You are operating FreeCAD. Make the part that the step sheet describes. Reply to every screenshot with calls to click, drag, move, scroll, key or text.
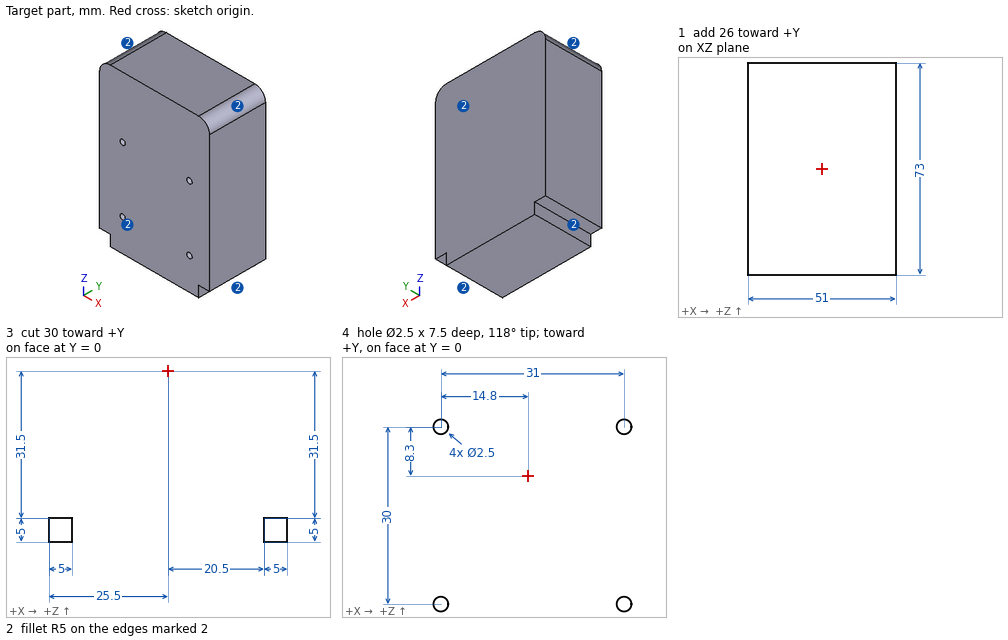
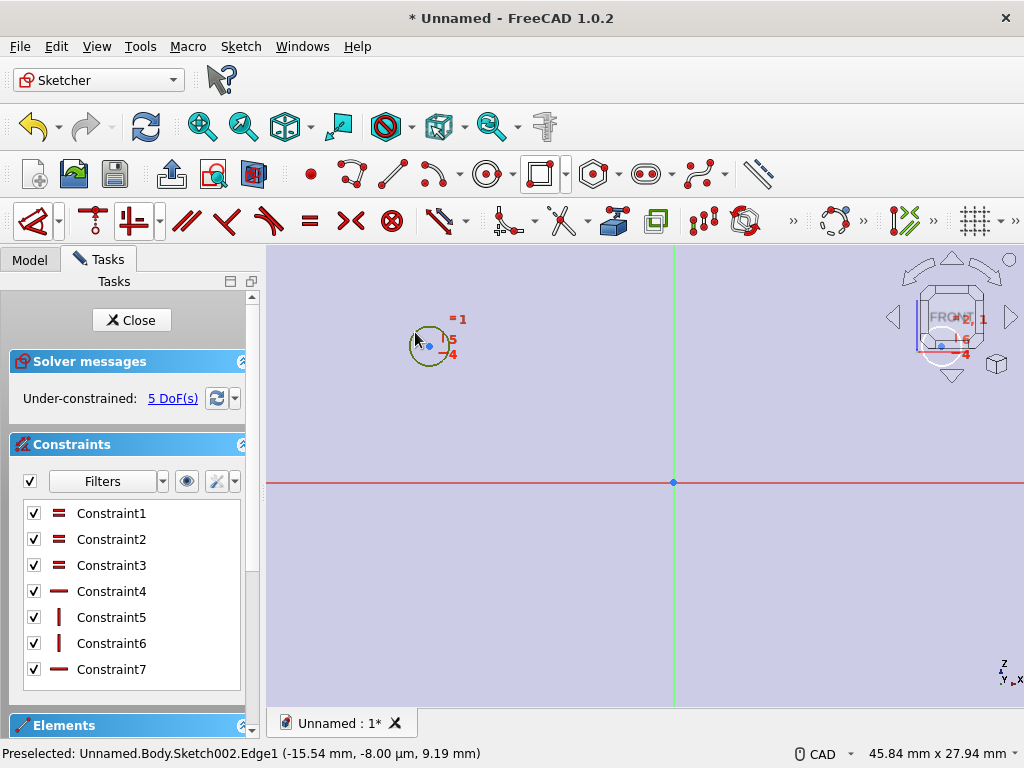
click(58, 222)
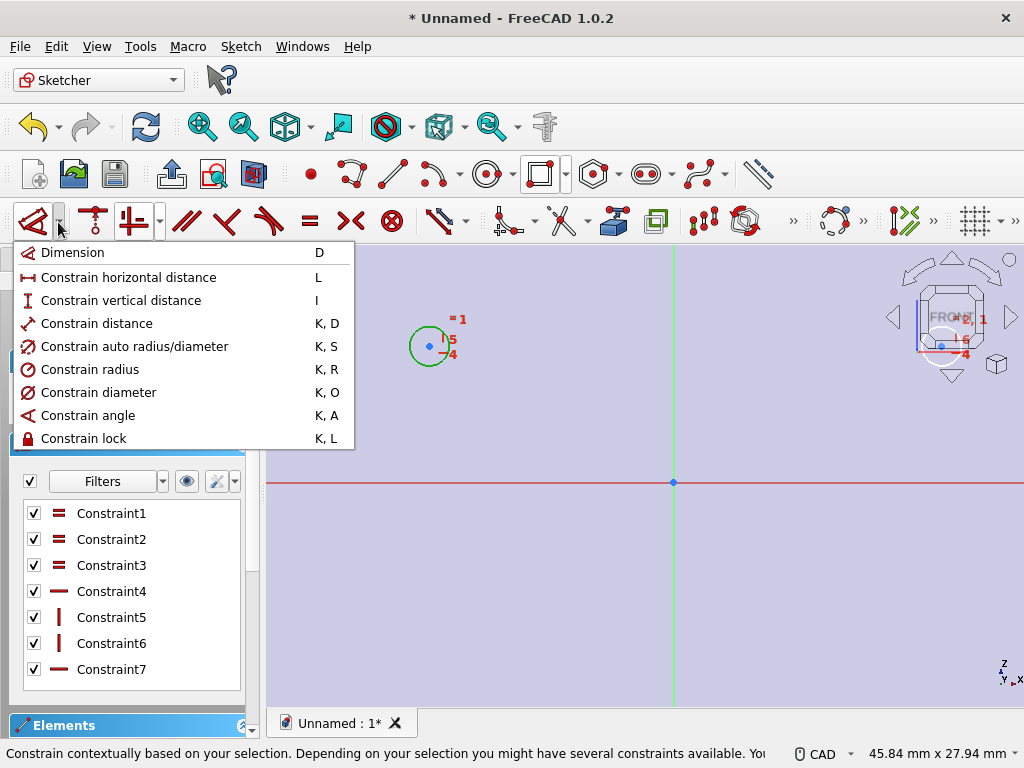
click(184, 392)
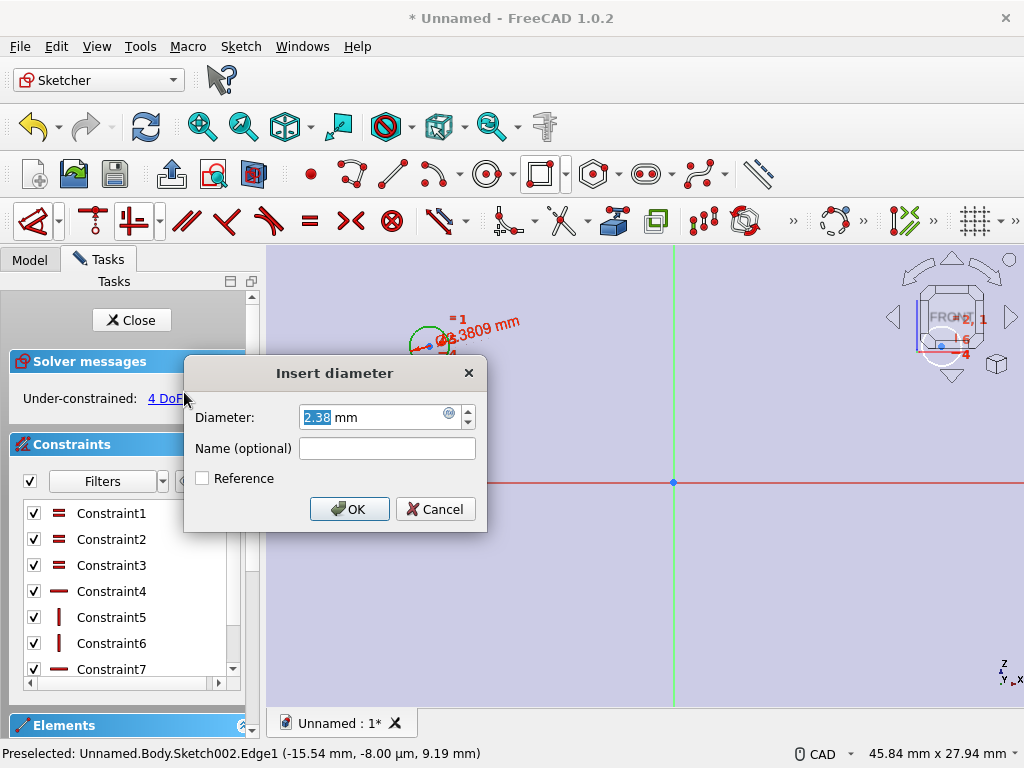
text(2.5)
key(Return)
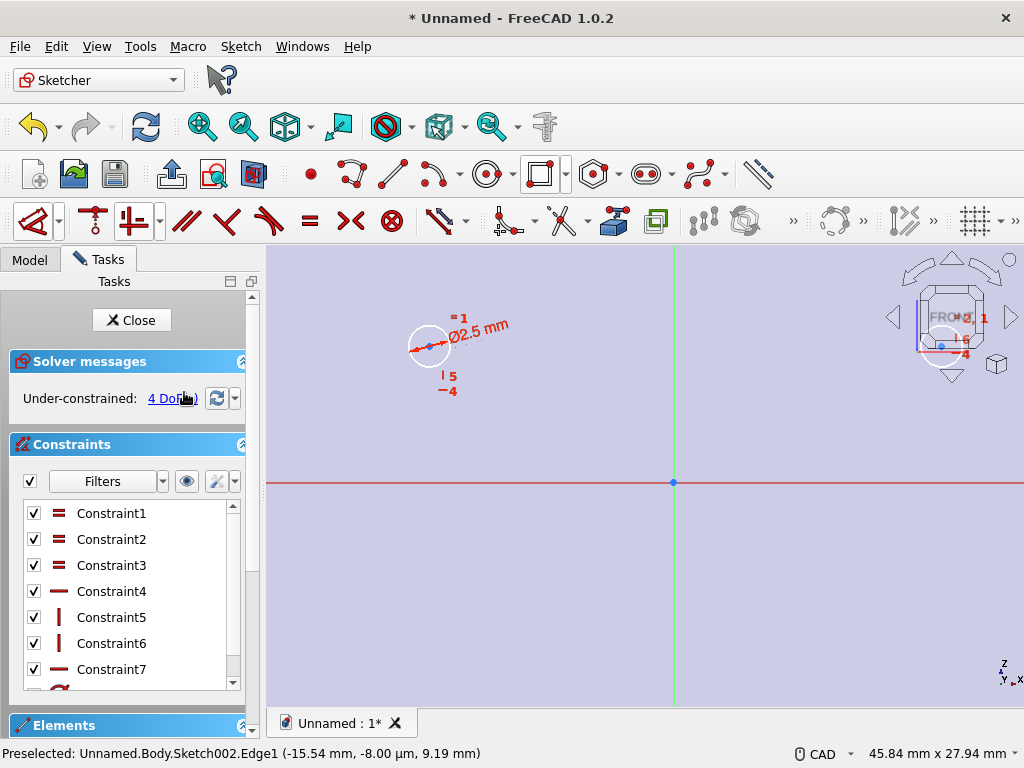
click(429, 346)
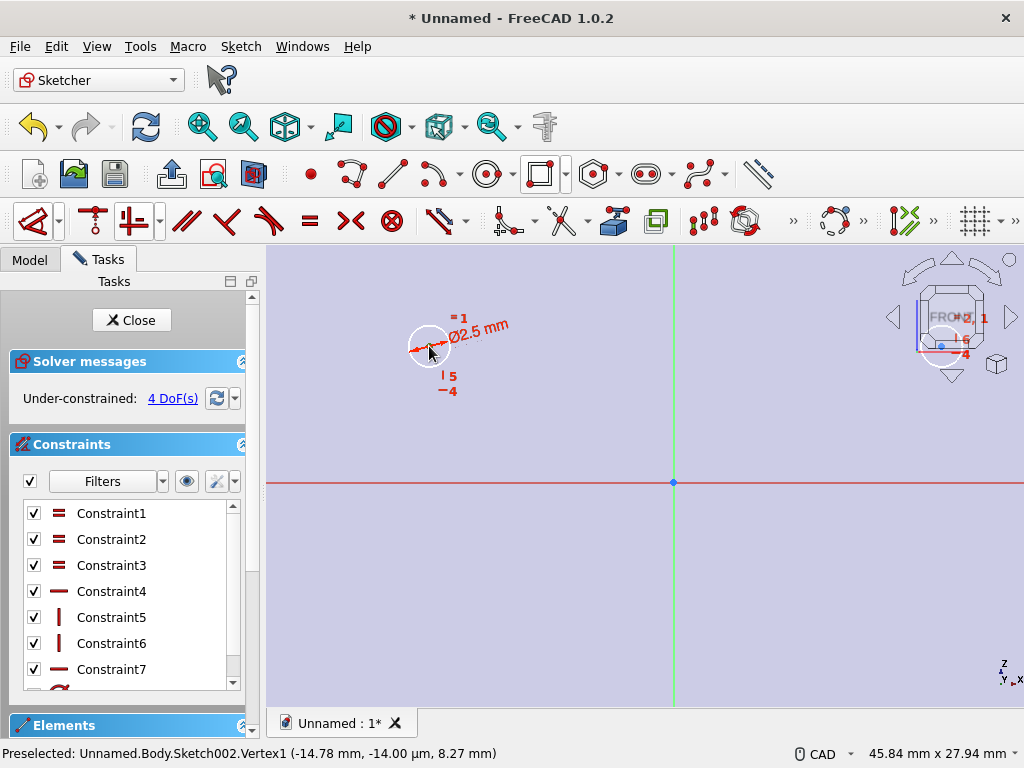
key(i)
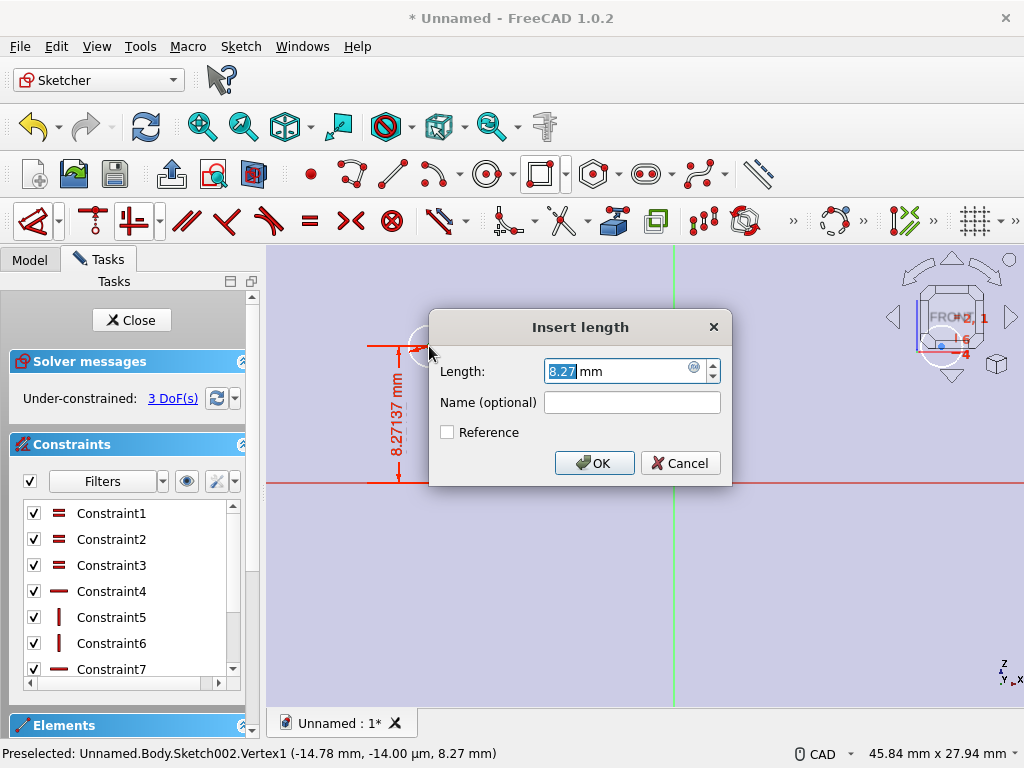
text(8.3)
key(Return)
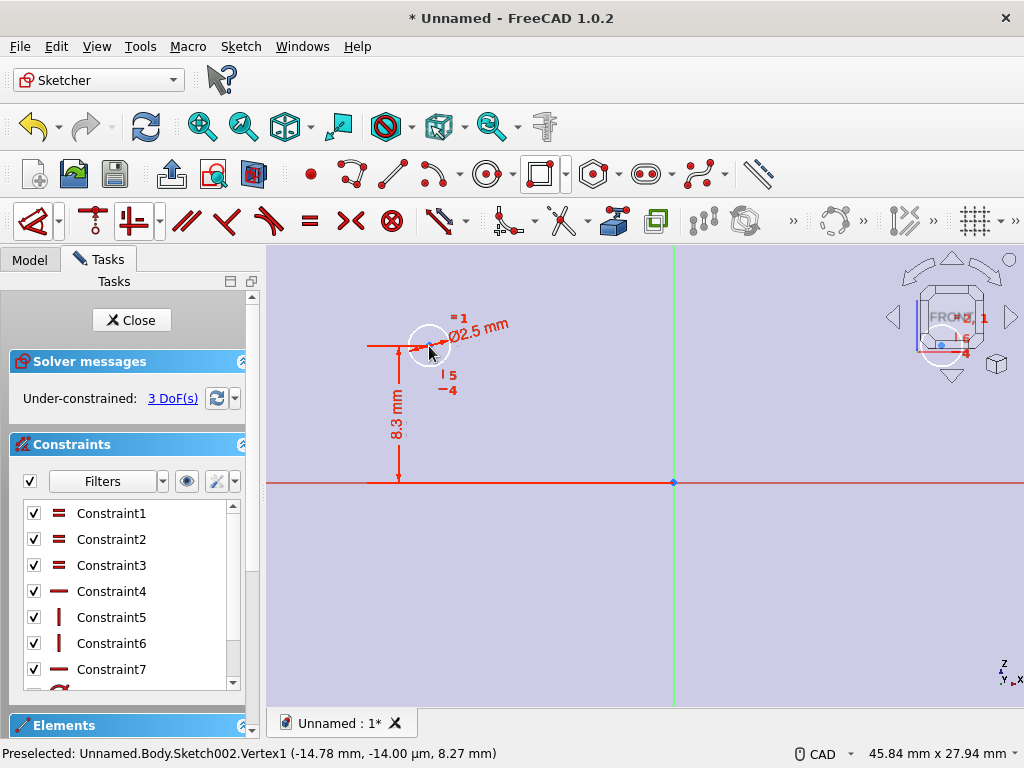
click(429, 346)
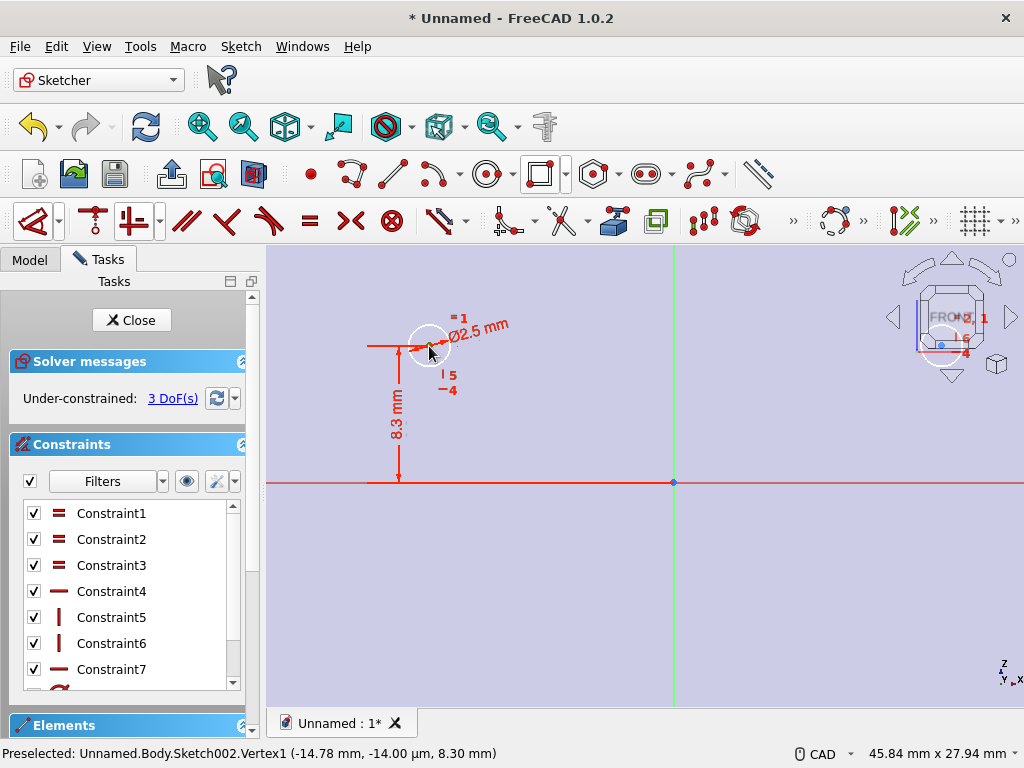
scroll(444, 333, down, 3)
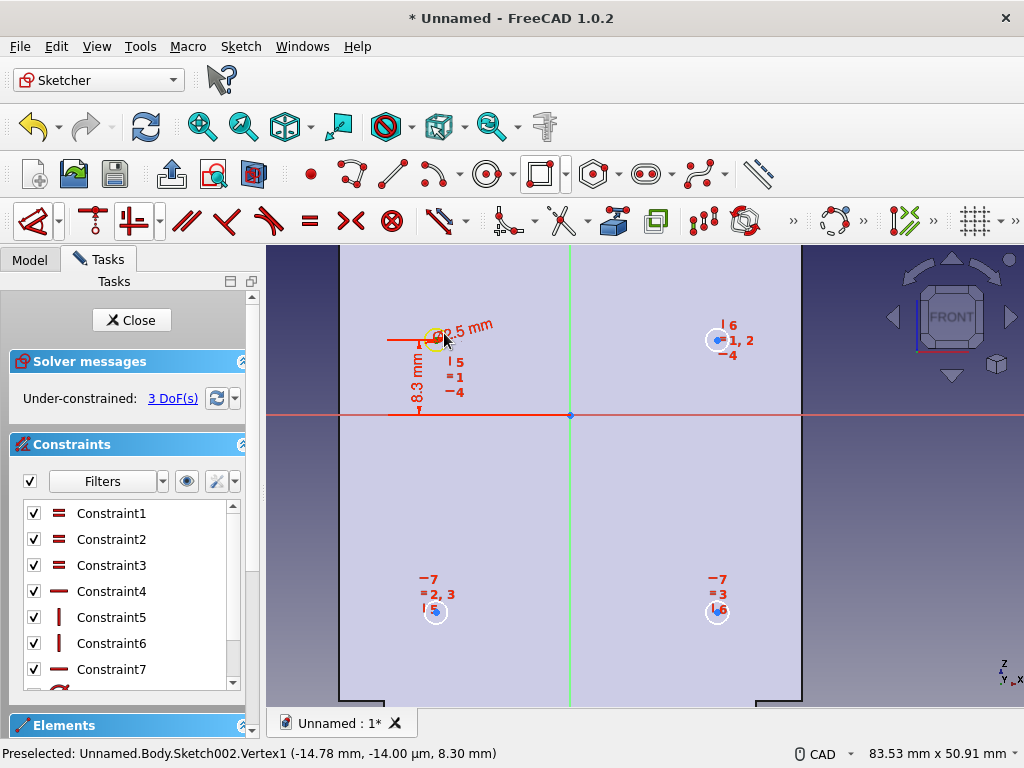
click(717, 340)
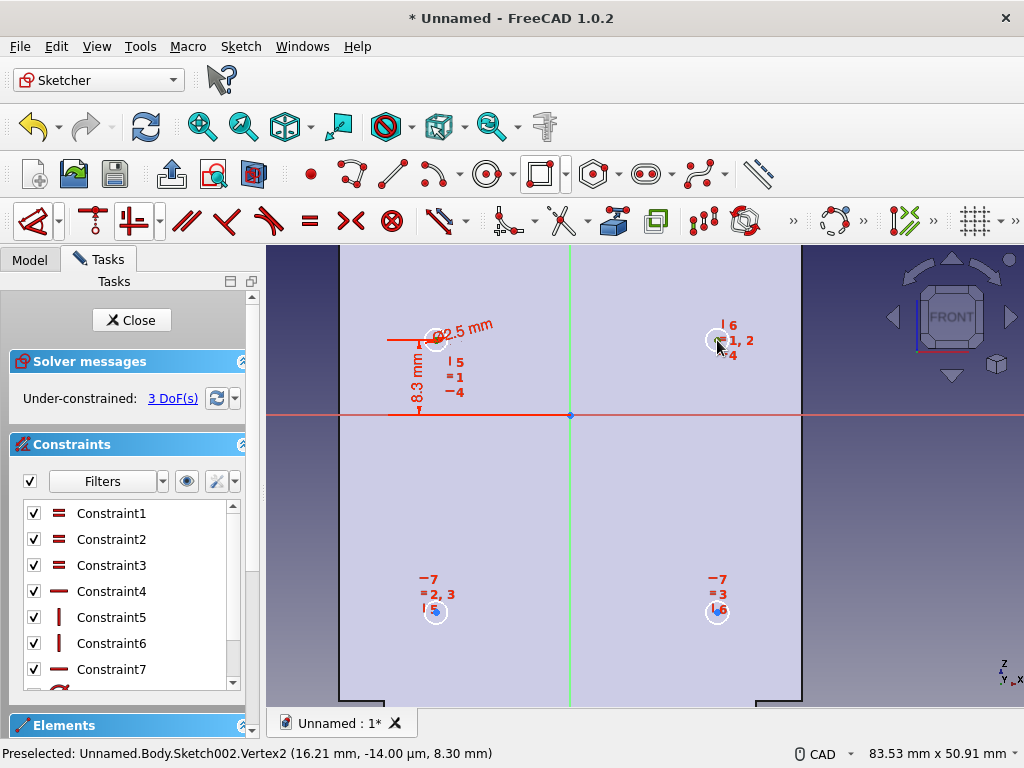
click(58, 222)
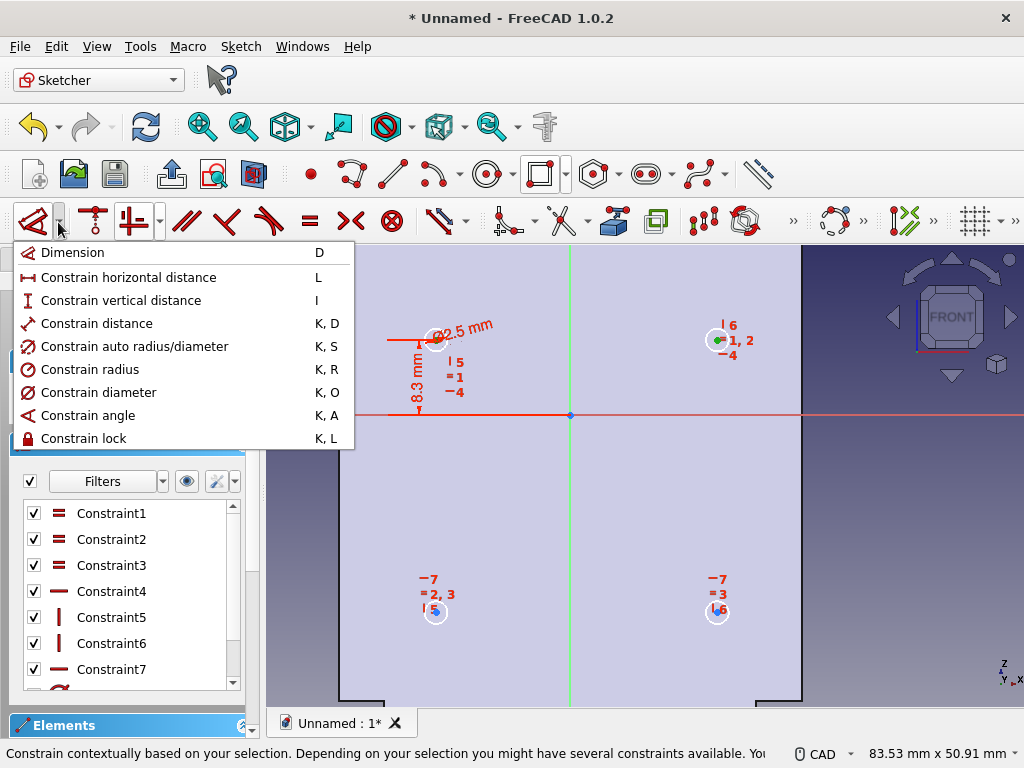
click(184, 278)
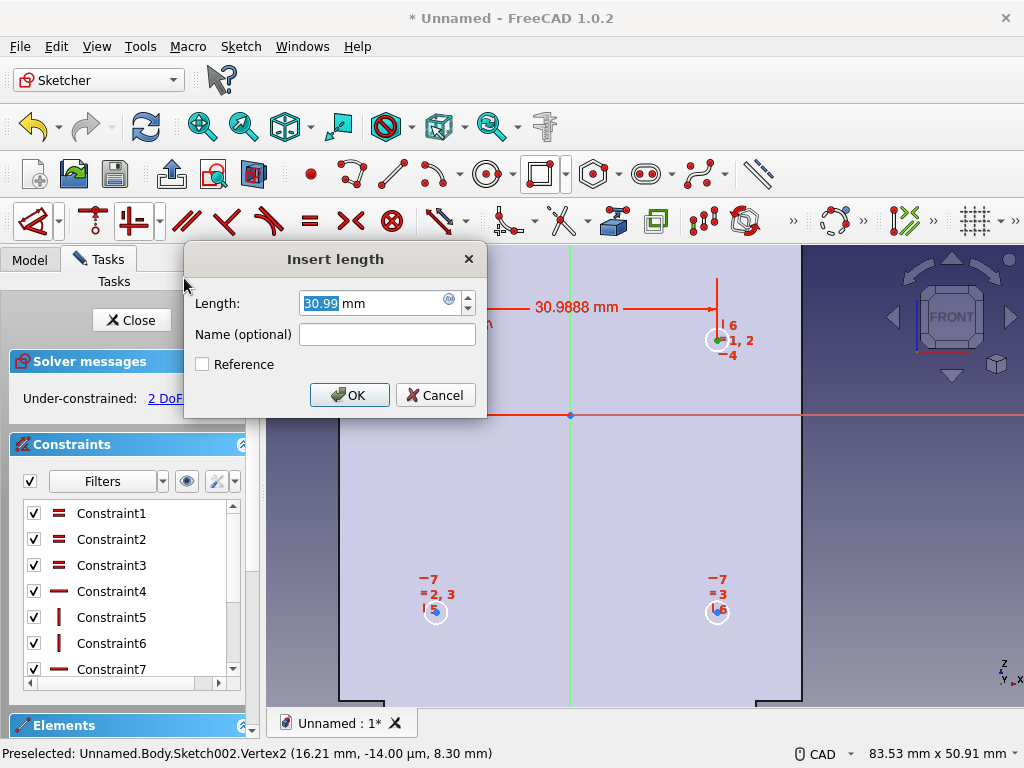
text(31)
key(Return)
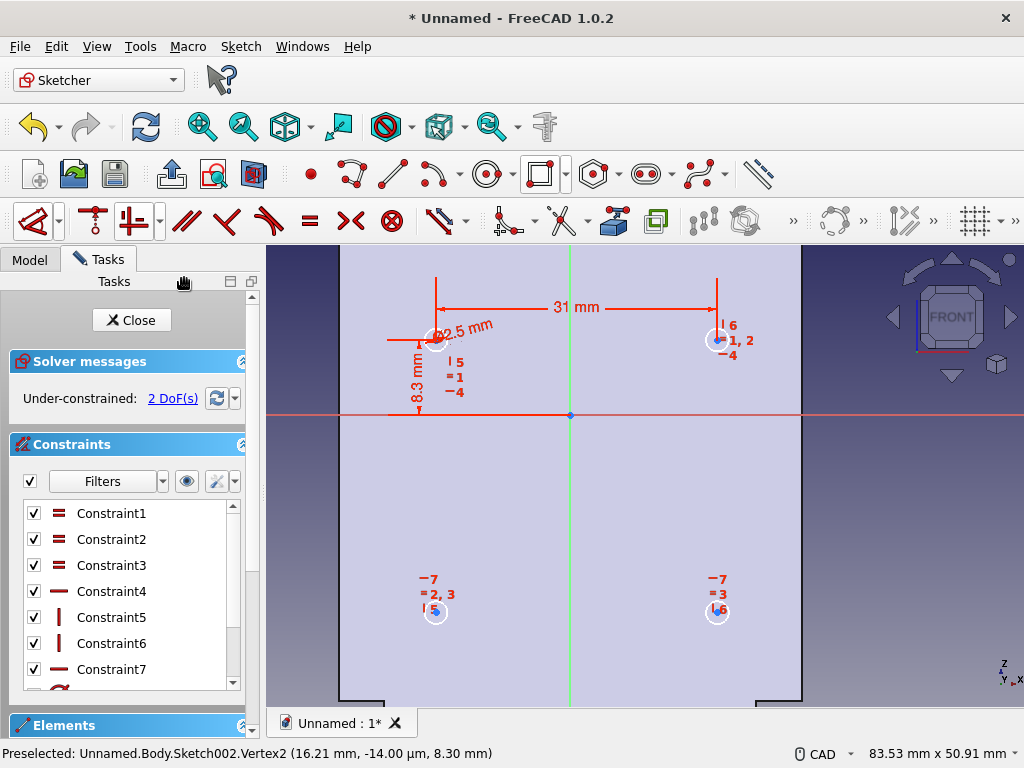
click(436, 340)